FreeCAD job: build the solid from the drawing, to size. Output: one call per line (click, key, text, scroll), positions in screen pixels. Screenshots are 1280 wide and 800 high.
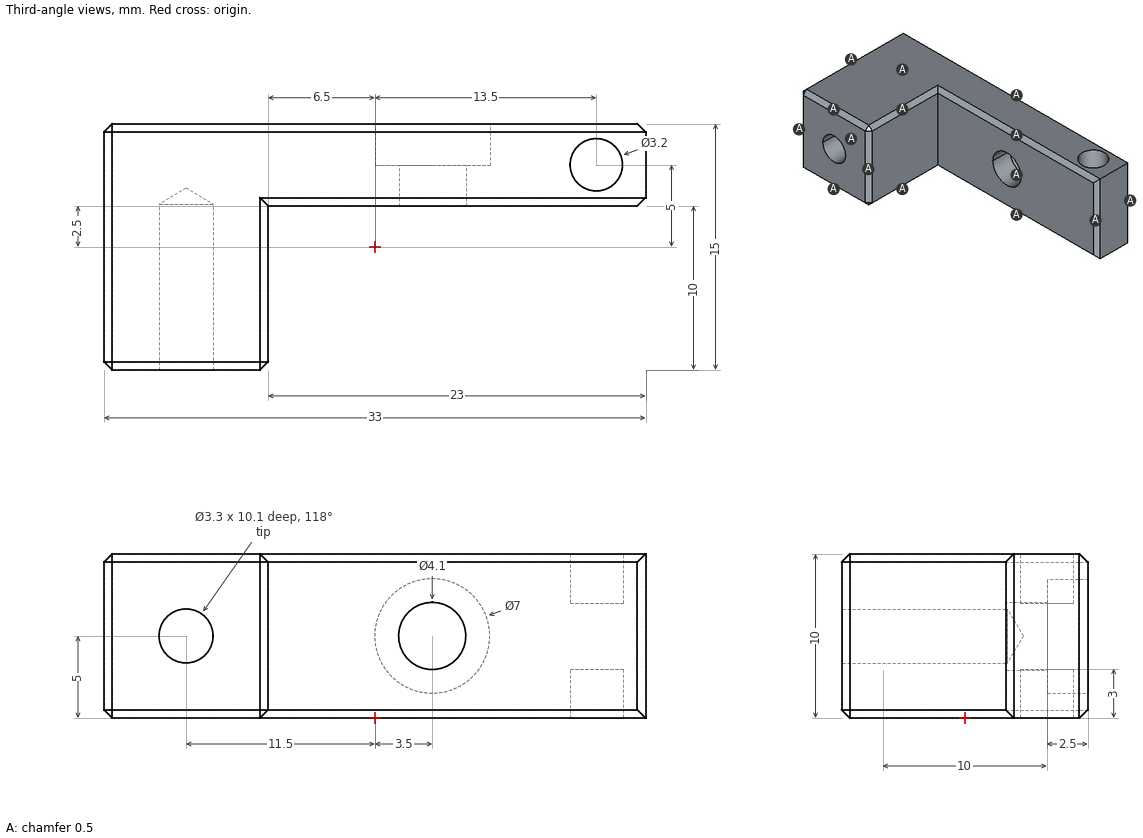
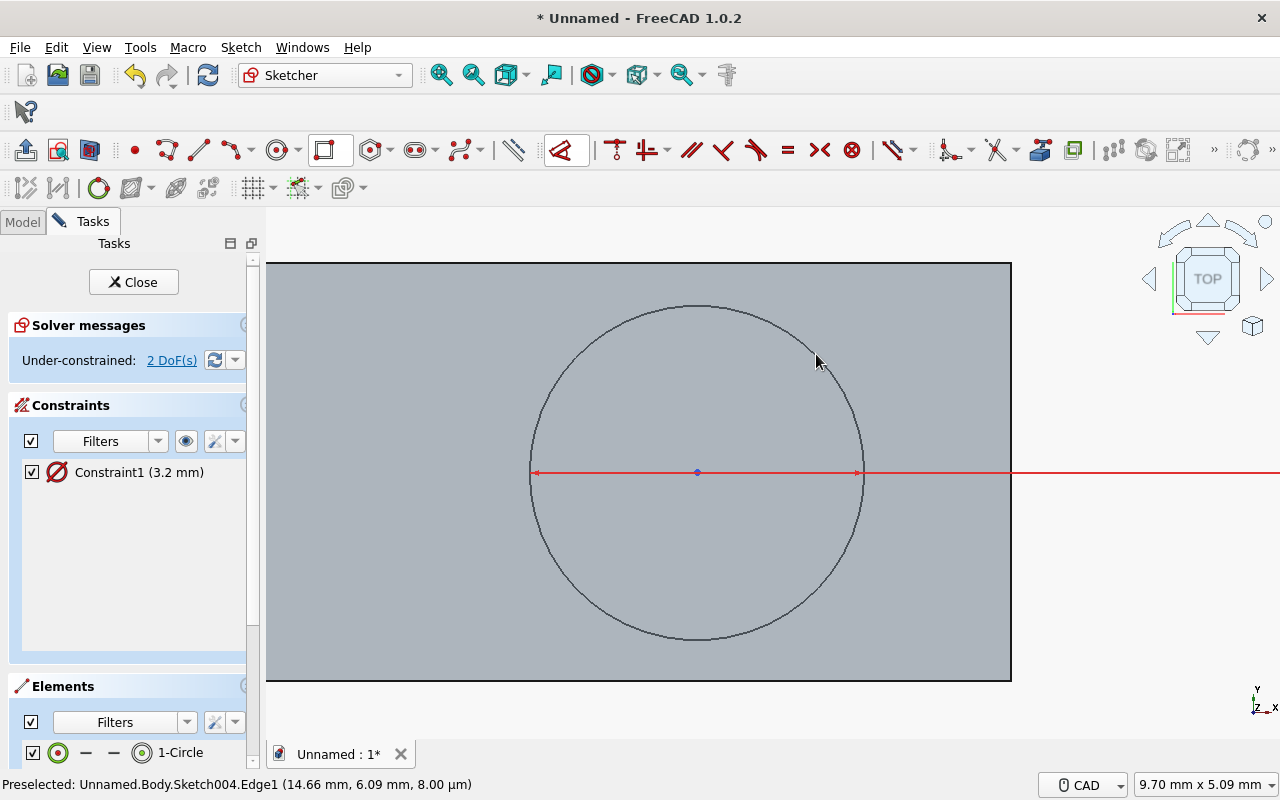
click(697, 473)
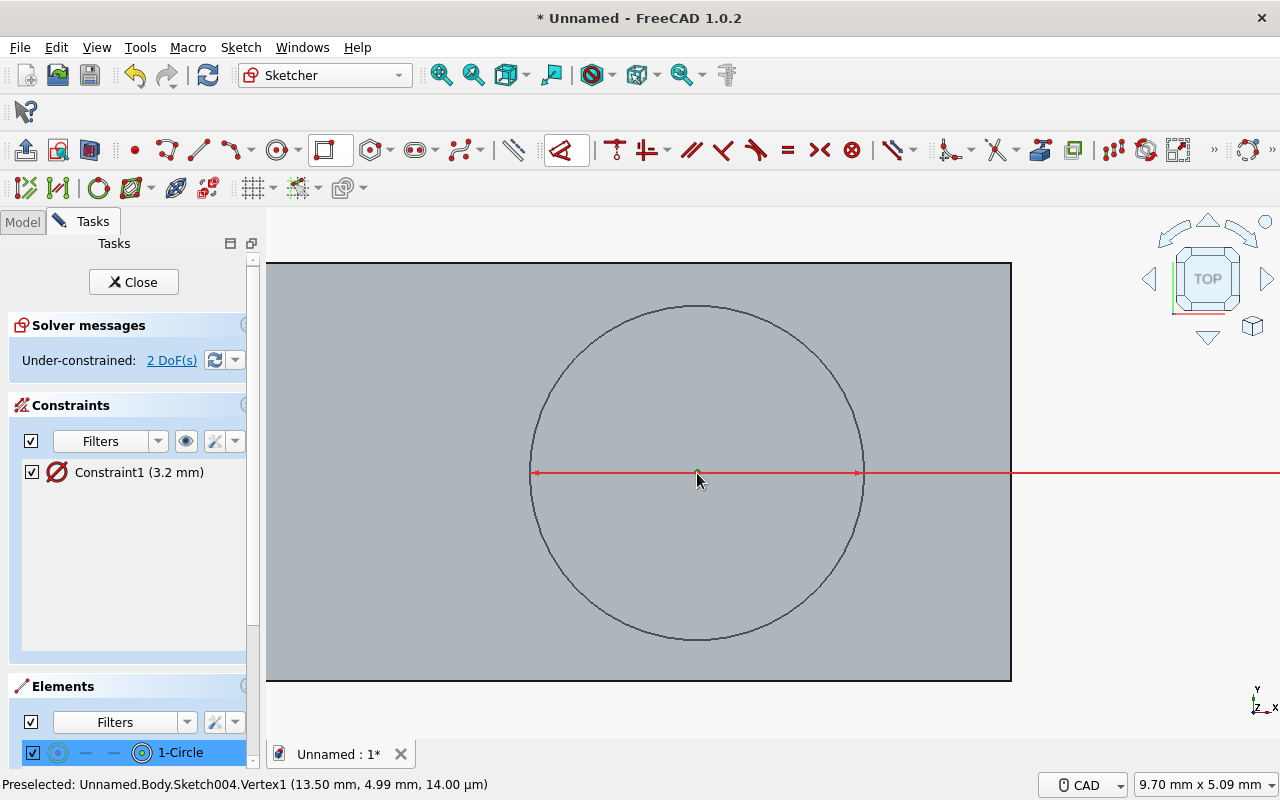
key(i)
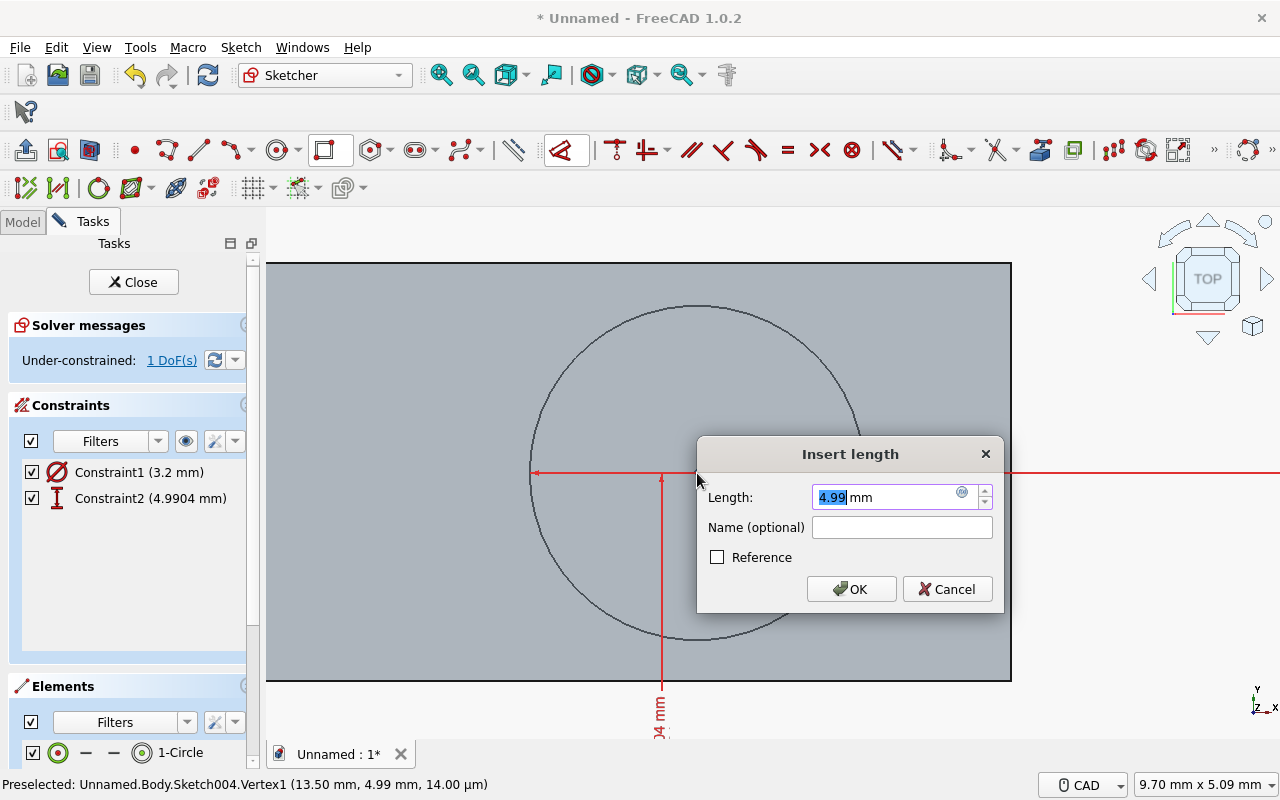
text(5)
key(Return)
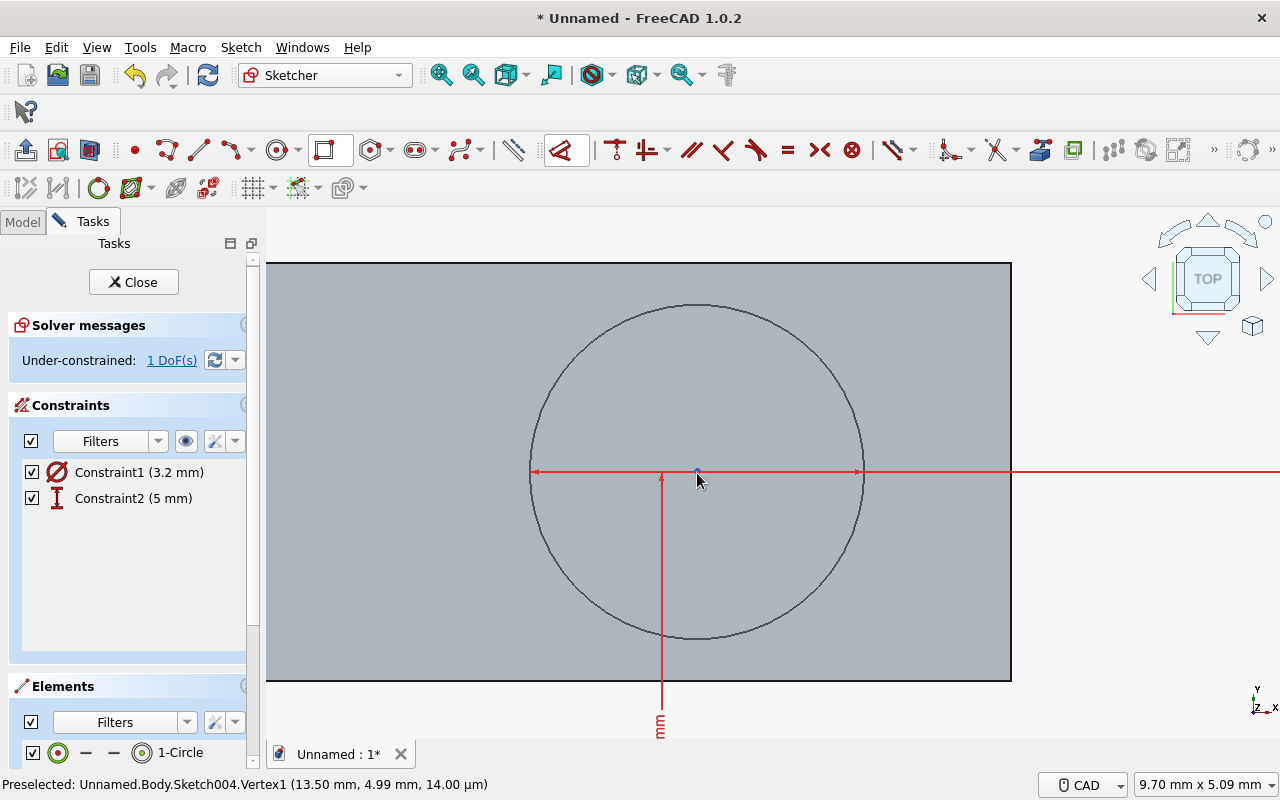
click(697, 472)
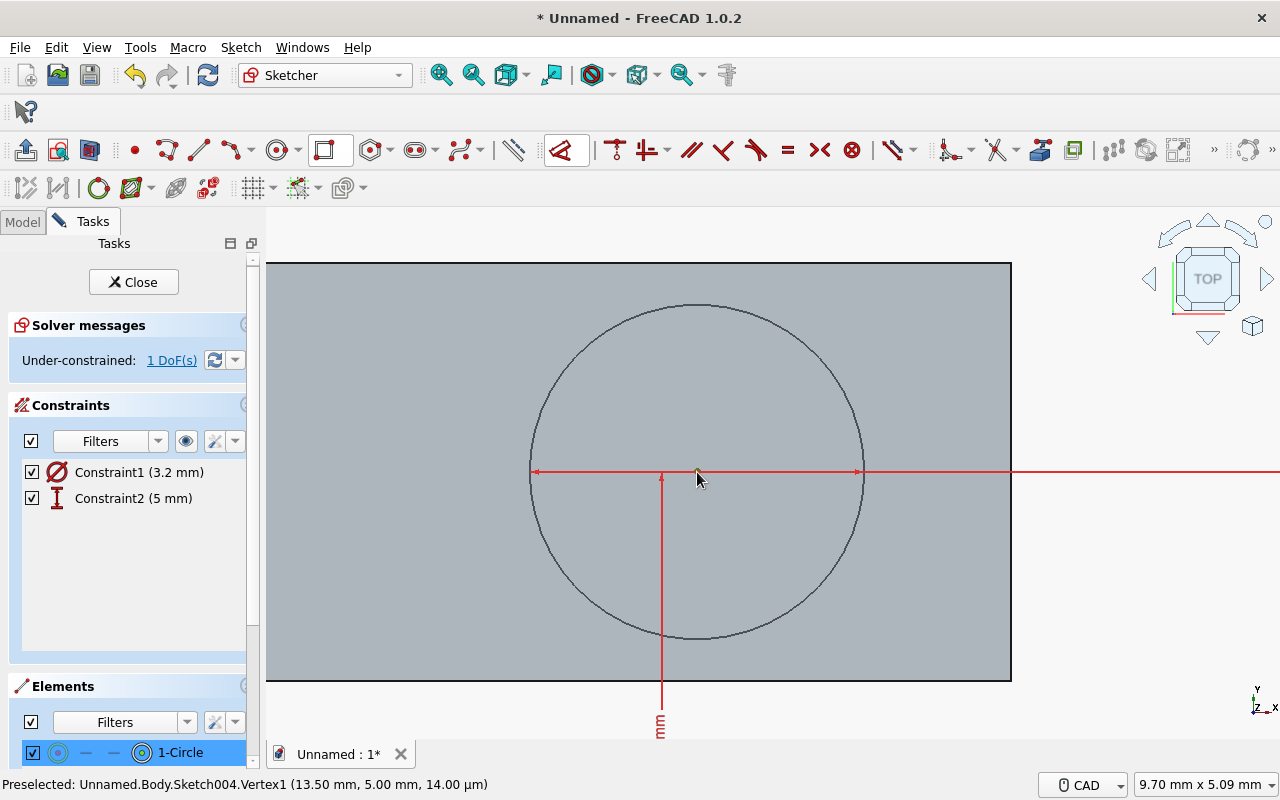
key(l)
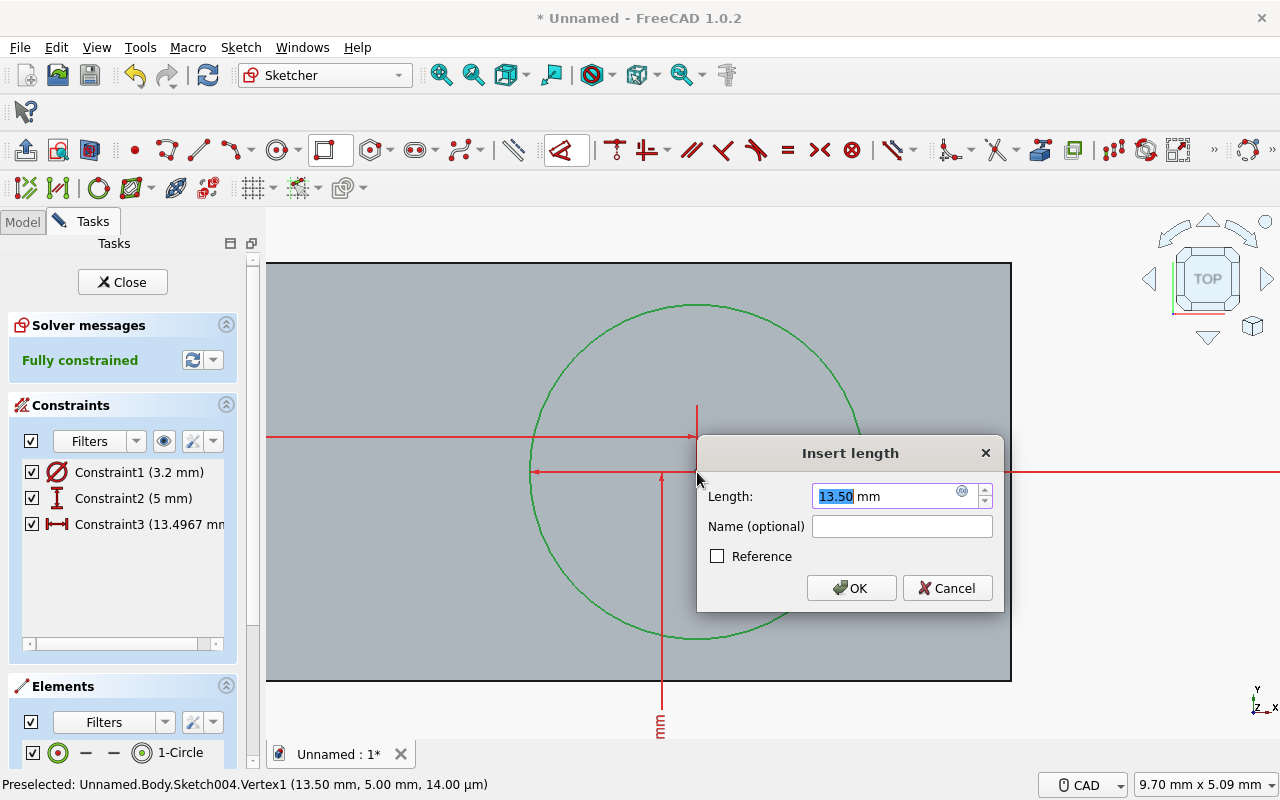
text(13.5)
key(Return)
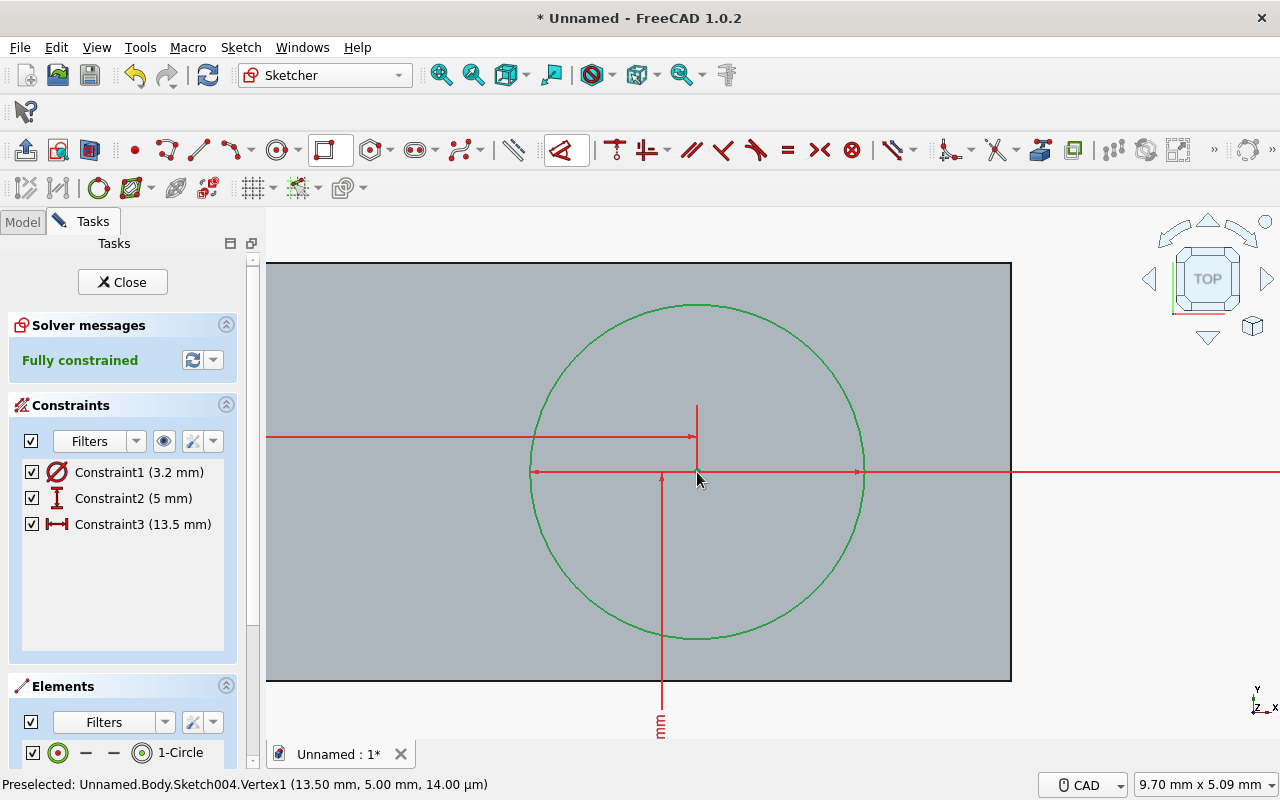
click(123, 282)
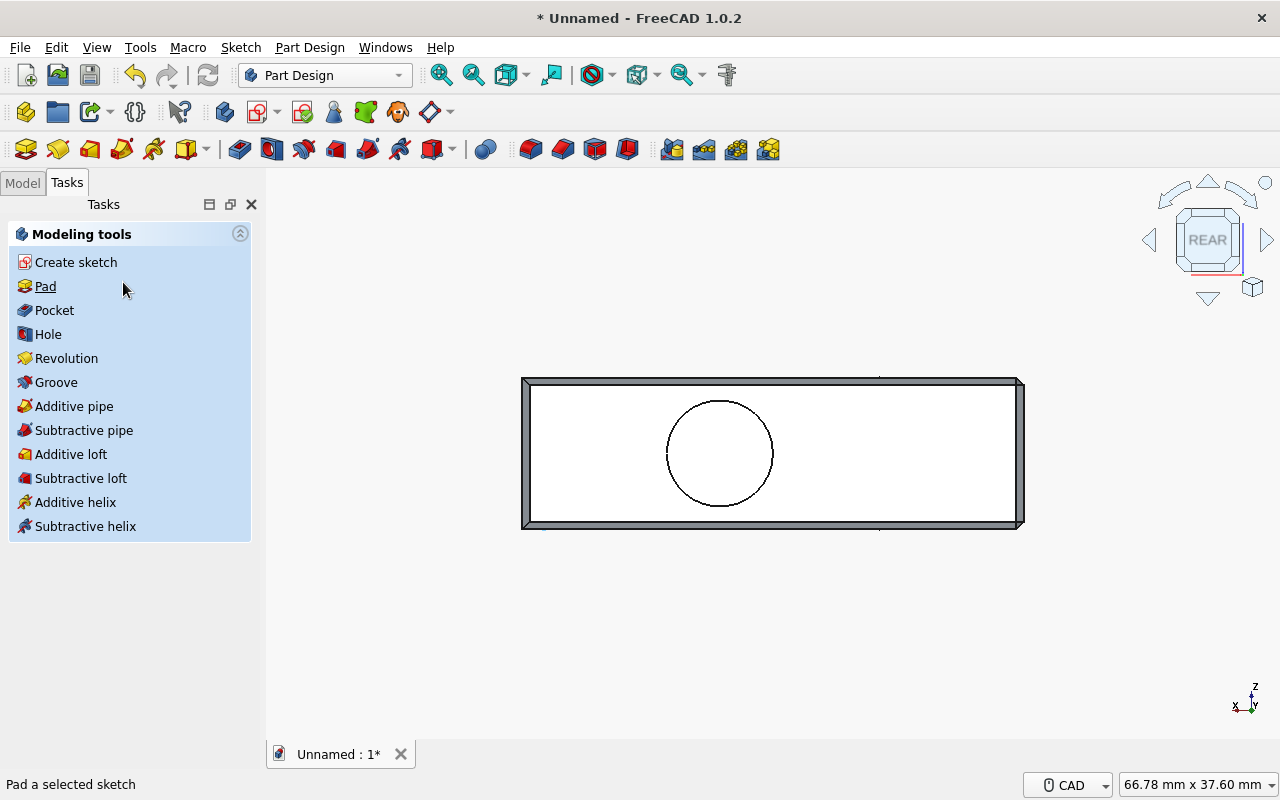
click(240, 150)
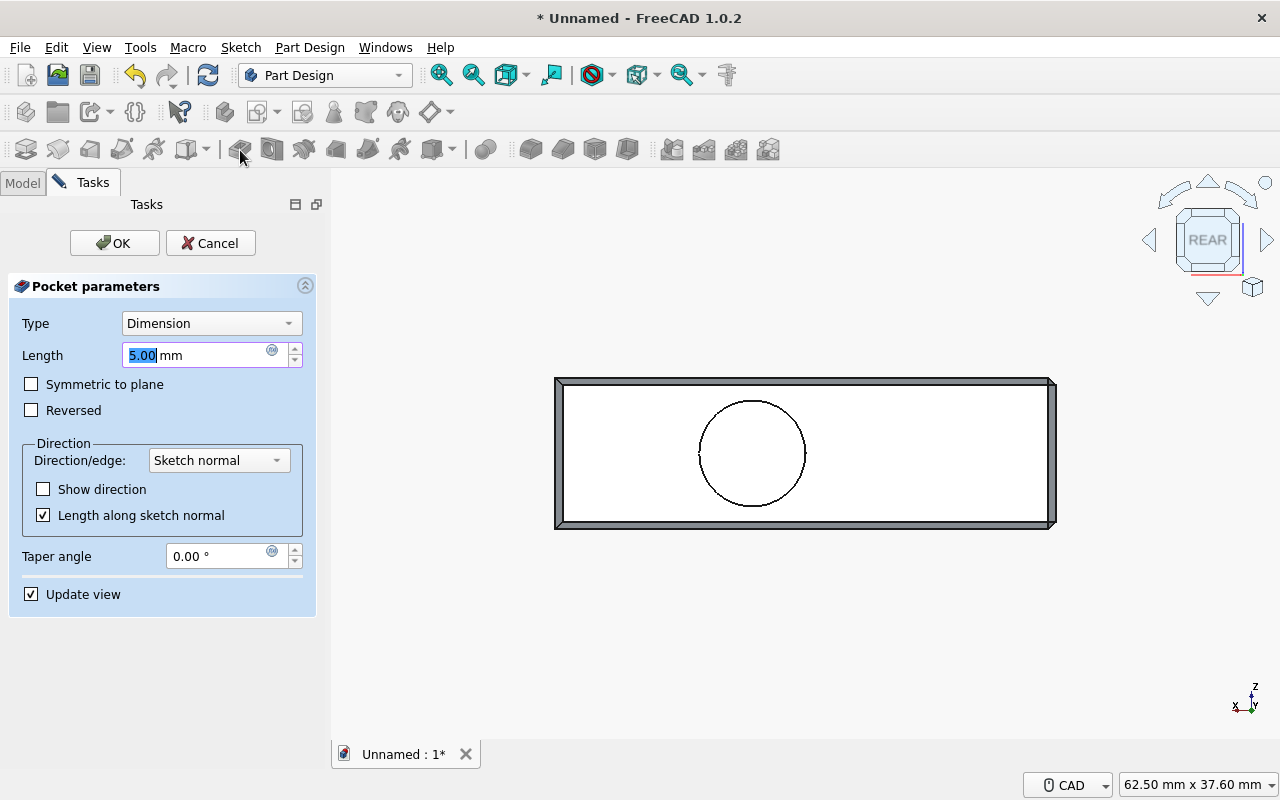
text(3)
key(Tab)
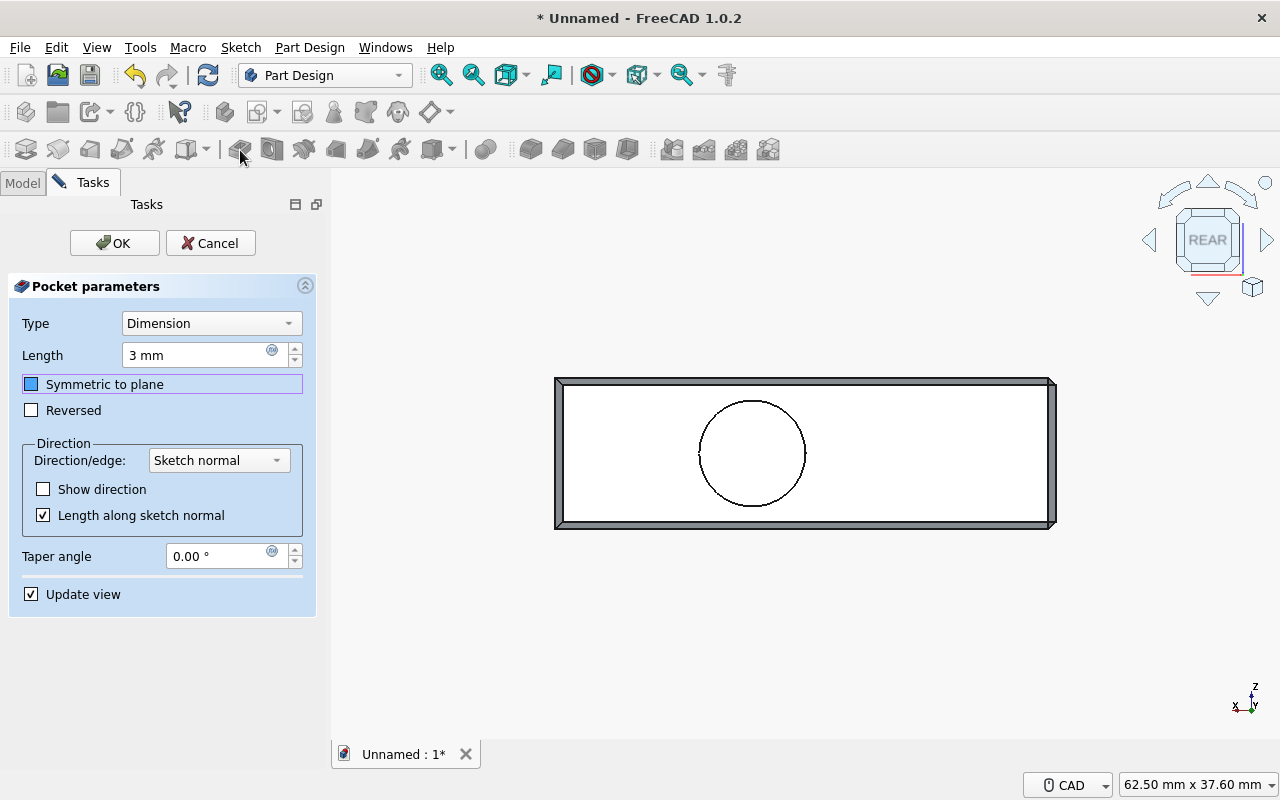
click(30, 410)